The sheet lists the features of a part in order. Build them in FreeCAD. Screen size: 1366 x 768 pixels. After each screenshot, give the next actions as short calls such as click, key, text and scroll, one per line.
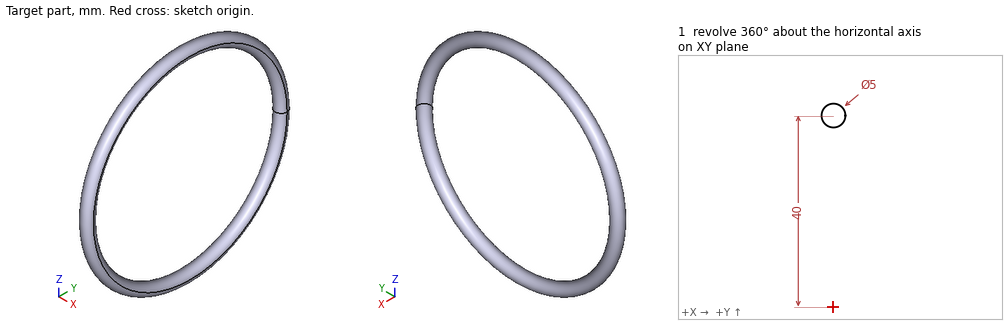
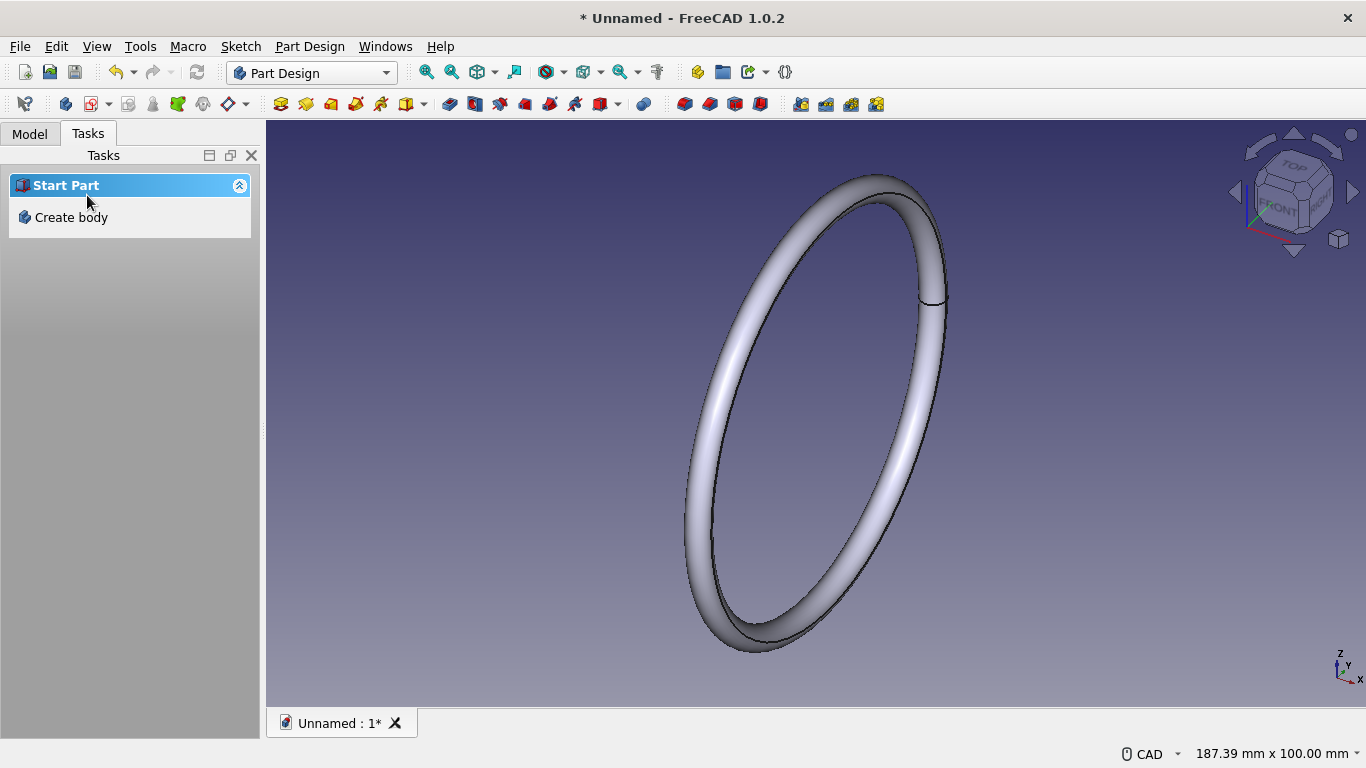
key(0)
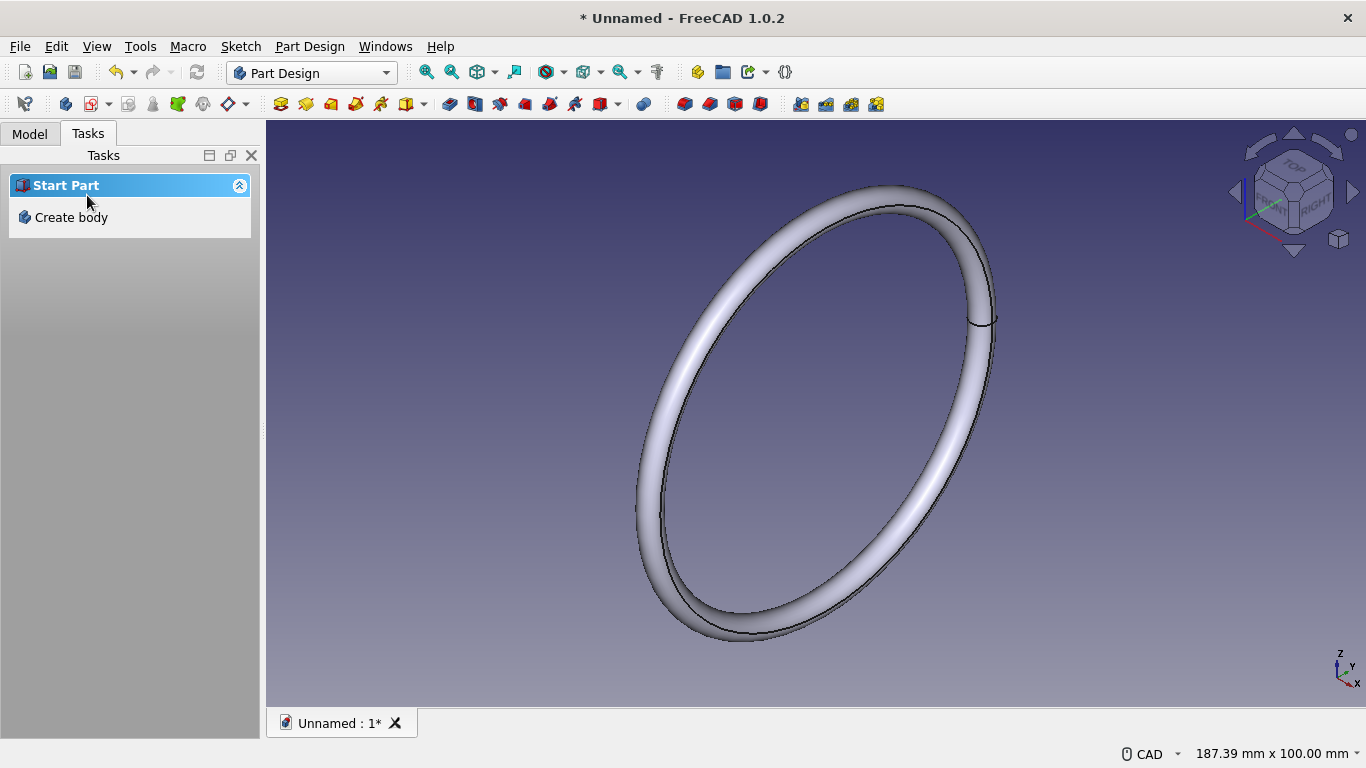
click(427, 72)